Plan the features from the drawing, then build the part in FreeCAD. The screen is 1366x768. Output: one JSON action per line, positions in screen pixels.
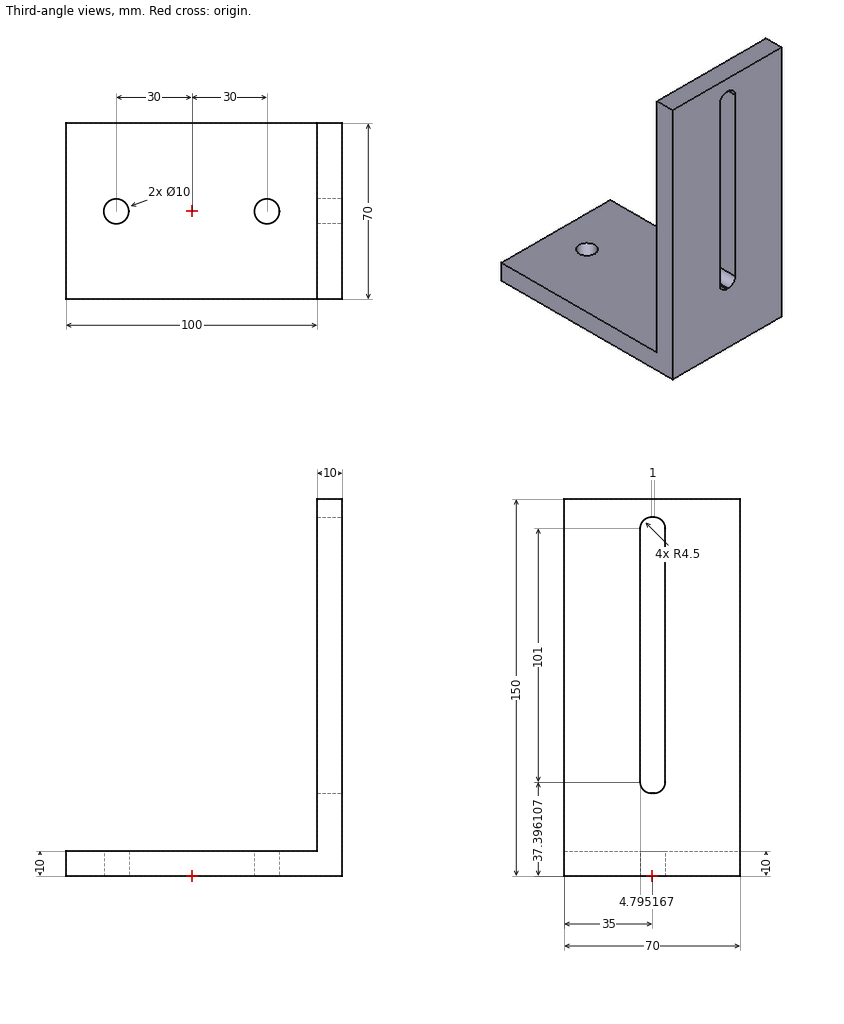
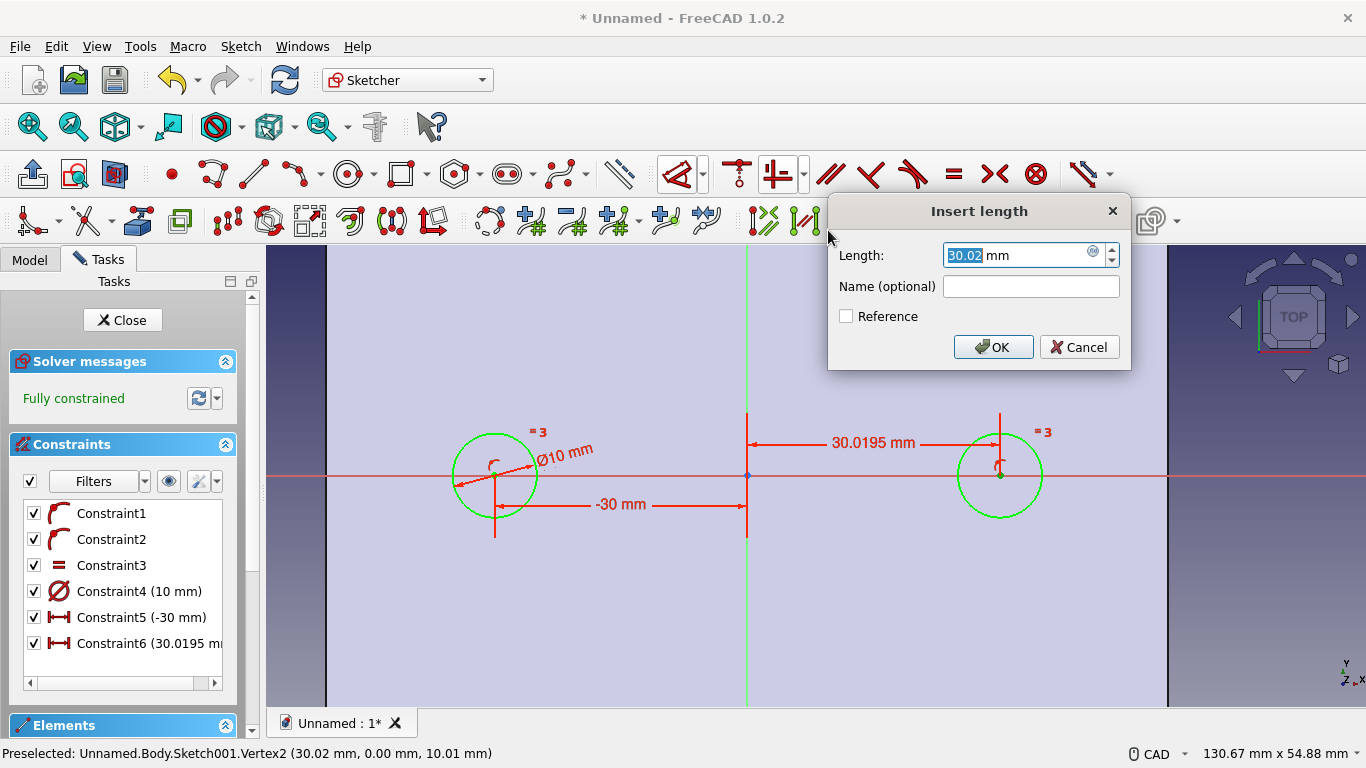
{"action": "type", "text": "30"}
{"action": "key", "text": "Return"}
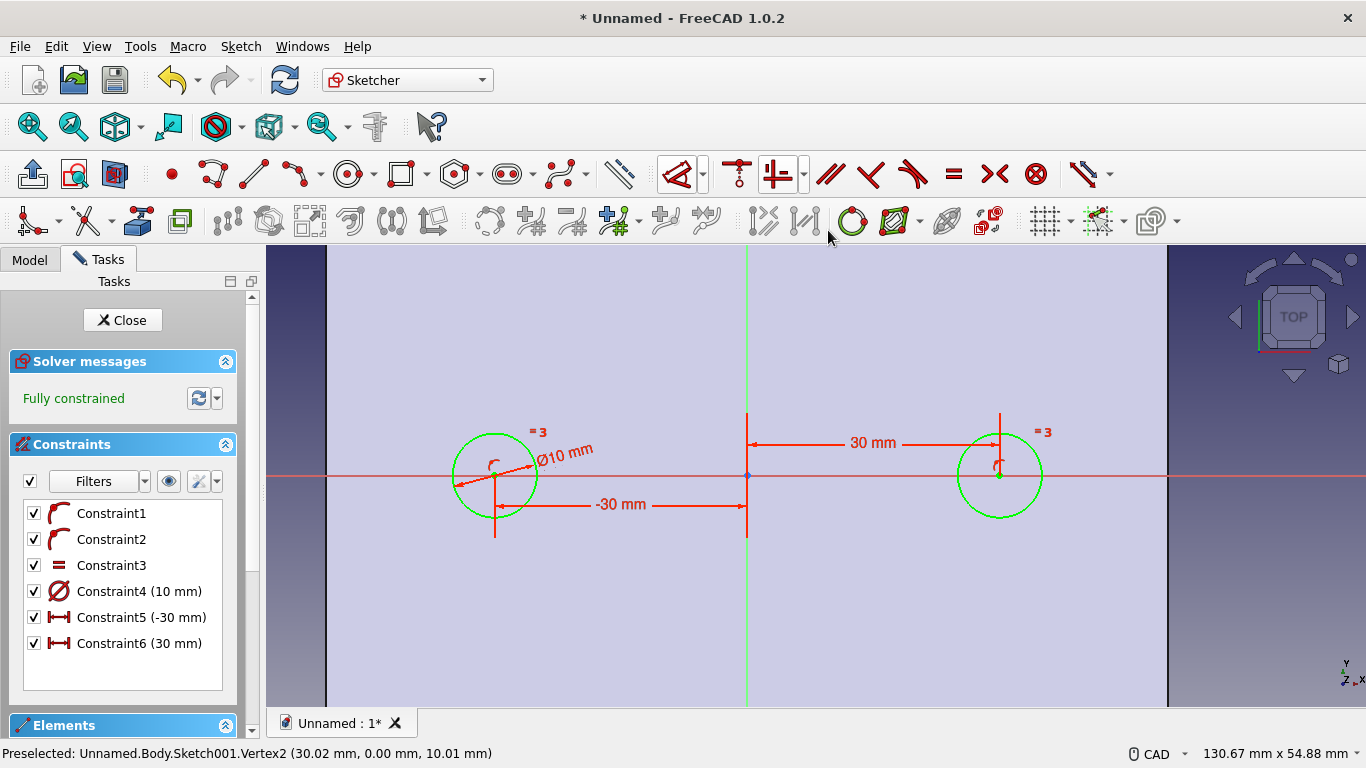
{"action": "left_click", "coordinate": [123, 320]}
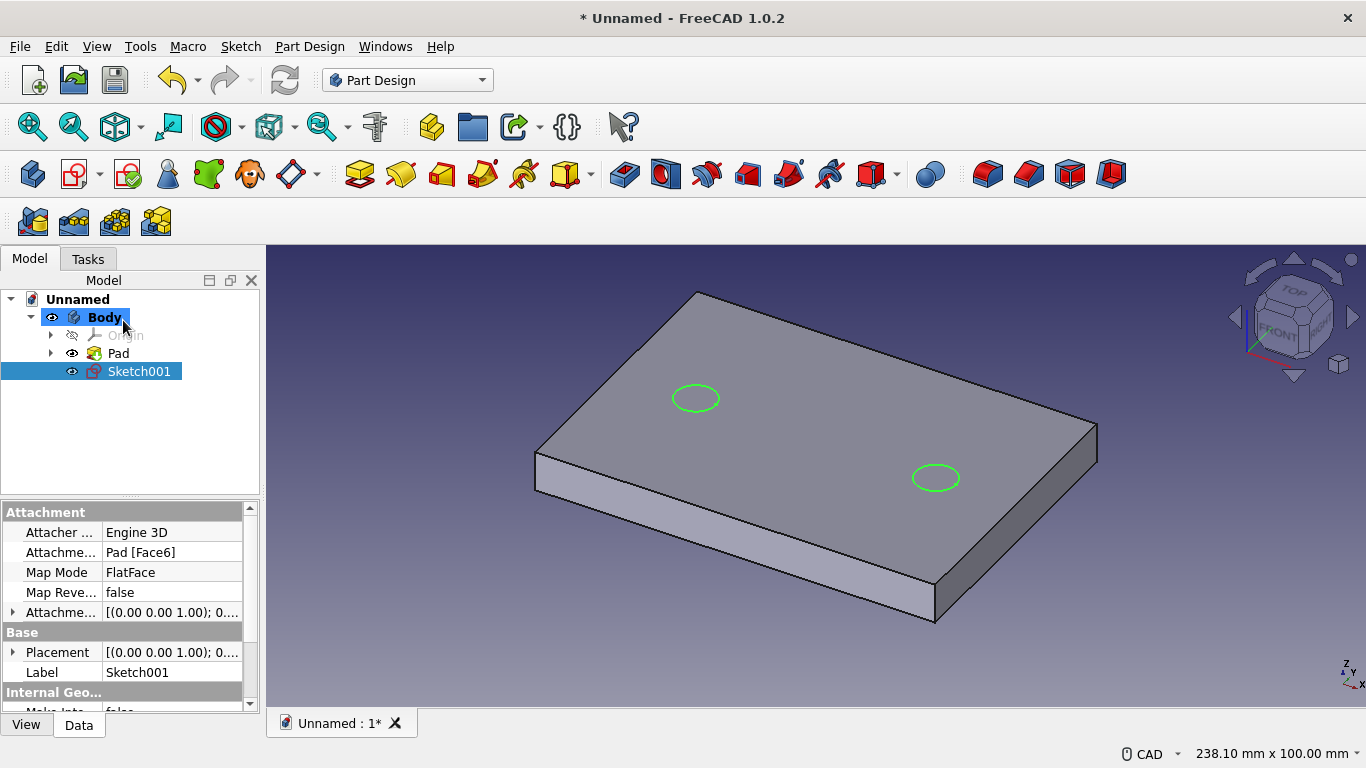
{"action": "left_click", "coordinate": [625, 174]}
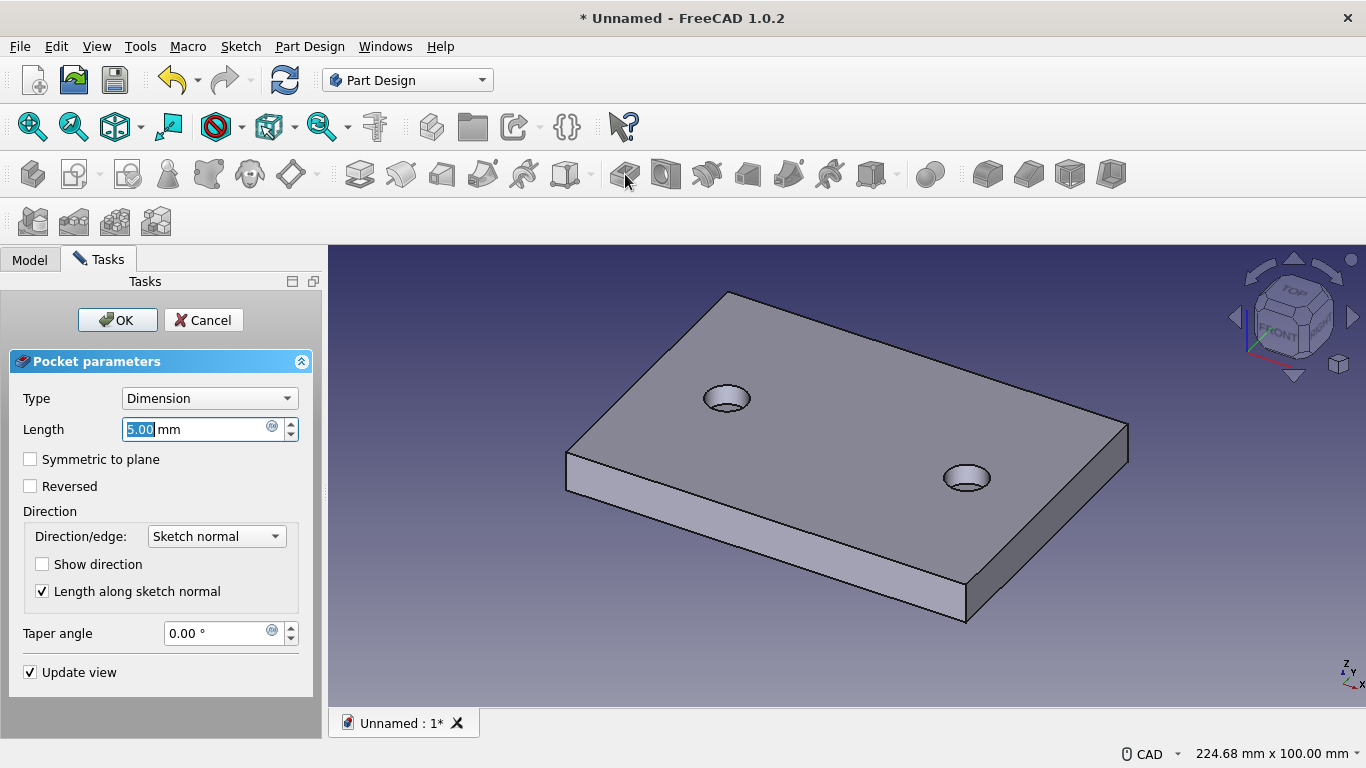
{"action": "type", "text": "10"}
{"action": "key", "text": "Tab"}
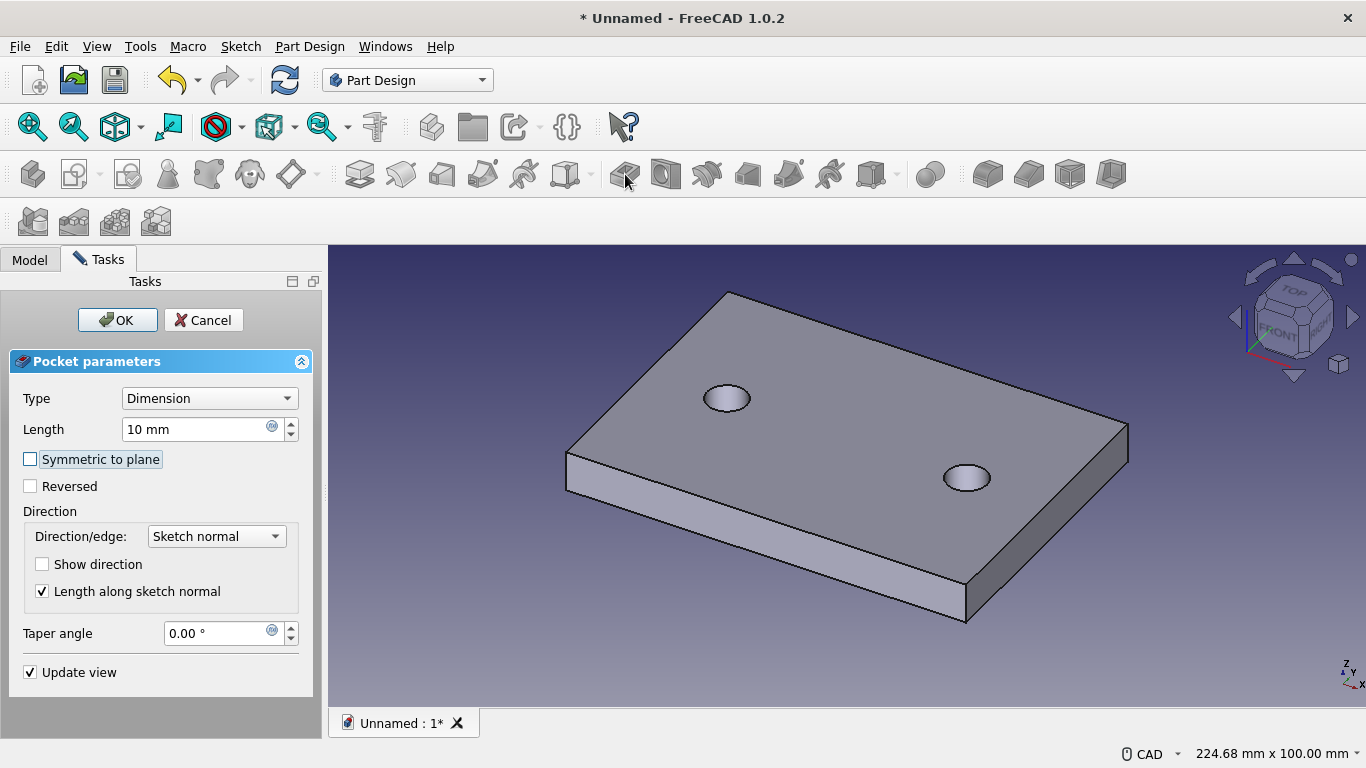
{"action": "left_click", "coordinate": [118, 320]}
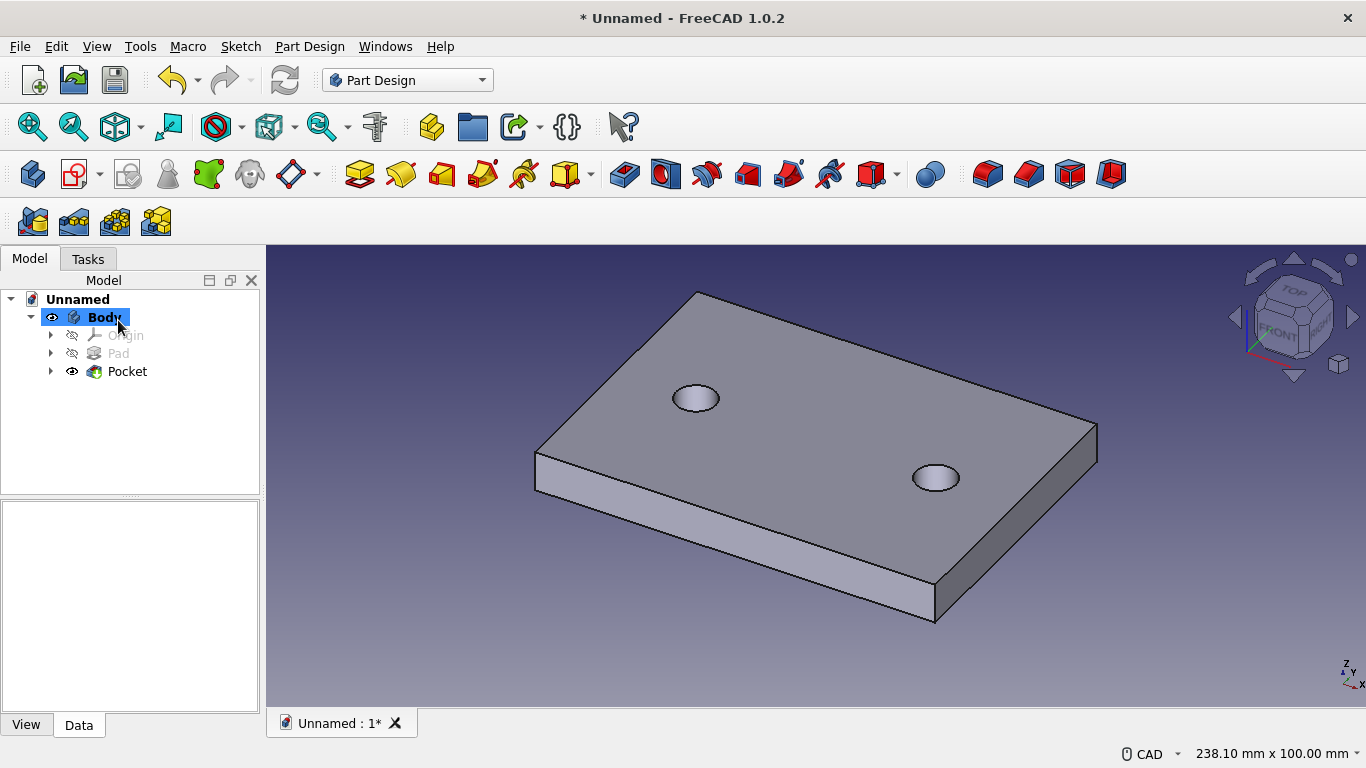
{"action": "left_click", "coordinate": [1085, 453]}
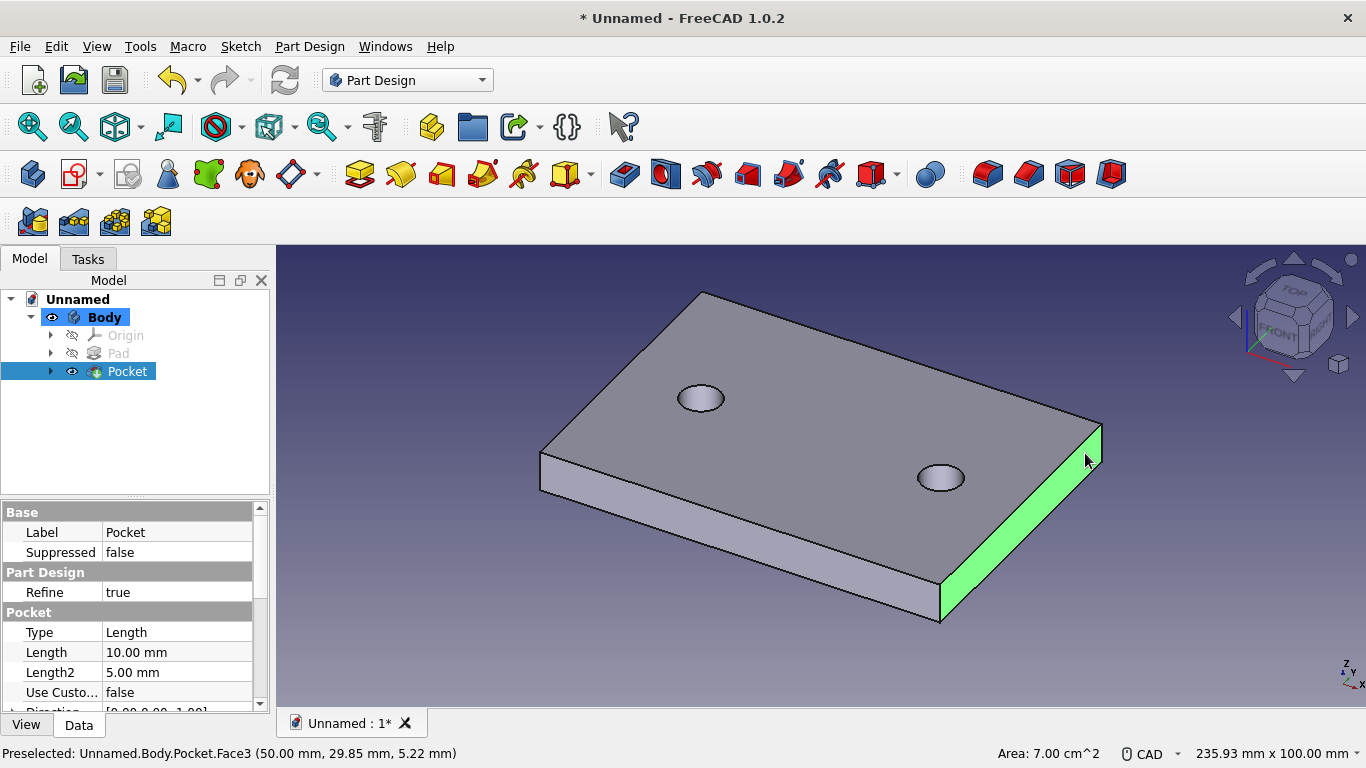
{"action": "left_click", "coordinate": [74, 174]}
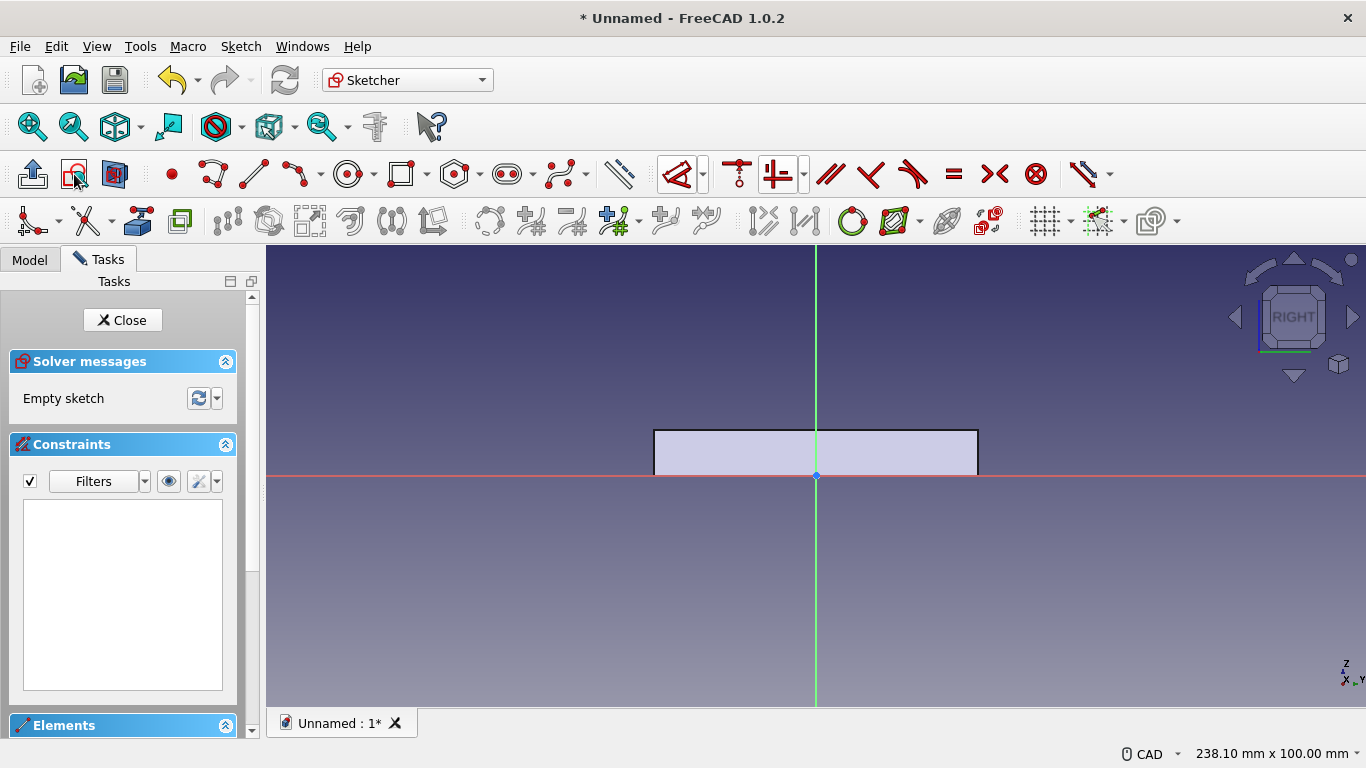
{"action": "scroll", "coordinate": [708, 678], "scroll_direction": "down", "scroll_amount": 5}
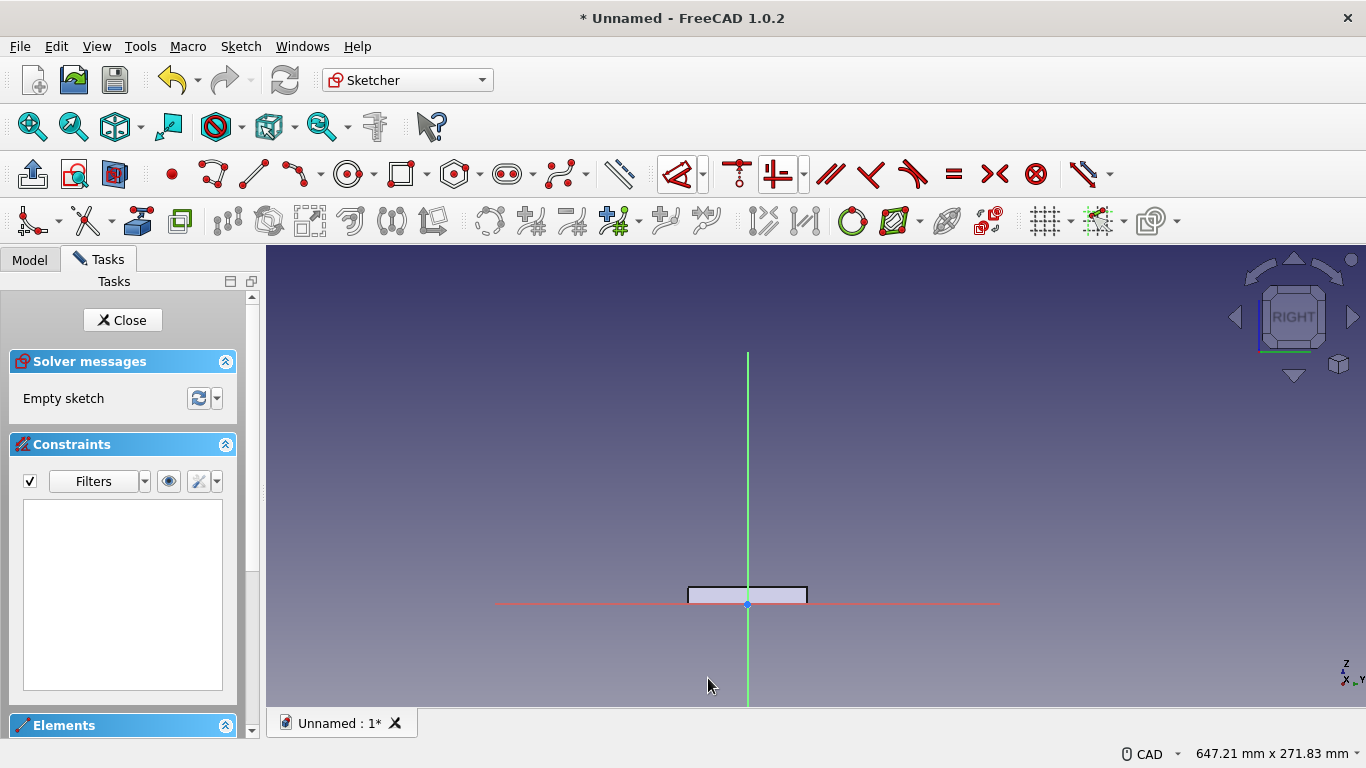
{"action": "left_click", "coordinate": [400, 174]}